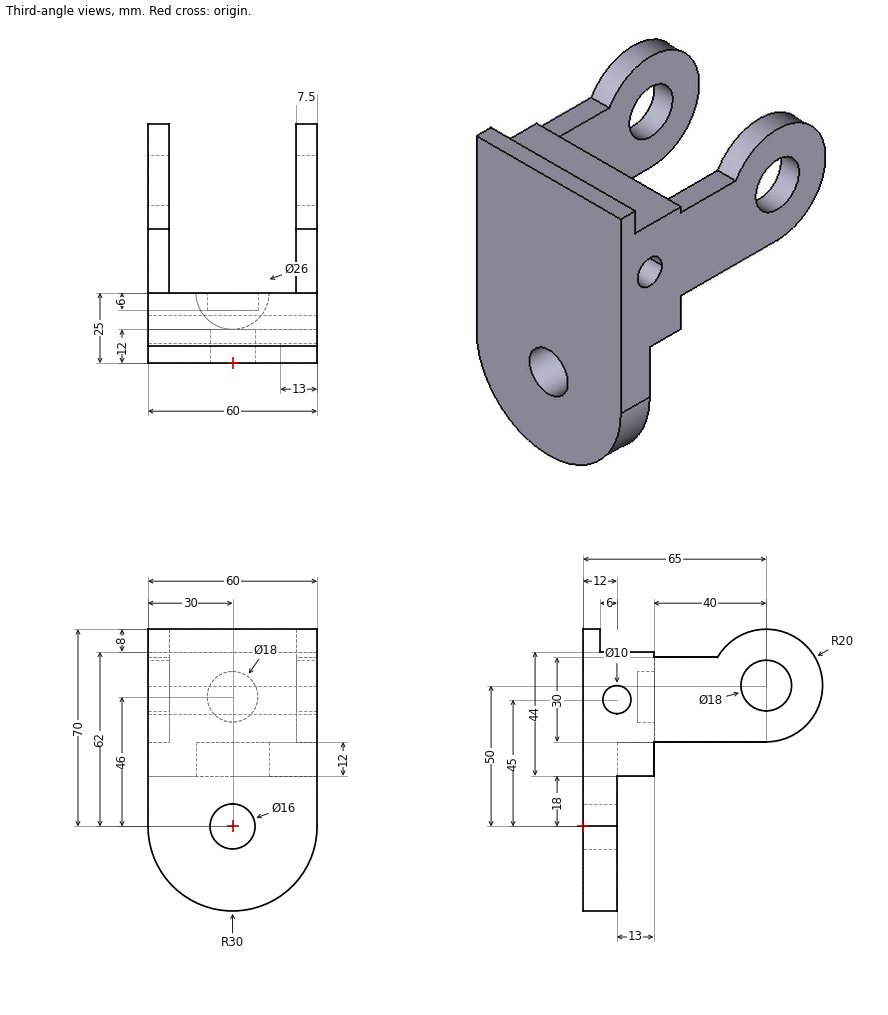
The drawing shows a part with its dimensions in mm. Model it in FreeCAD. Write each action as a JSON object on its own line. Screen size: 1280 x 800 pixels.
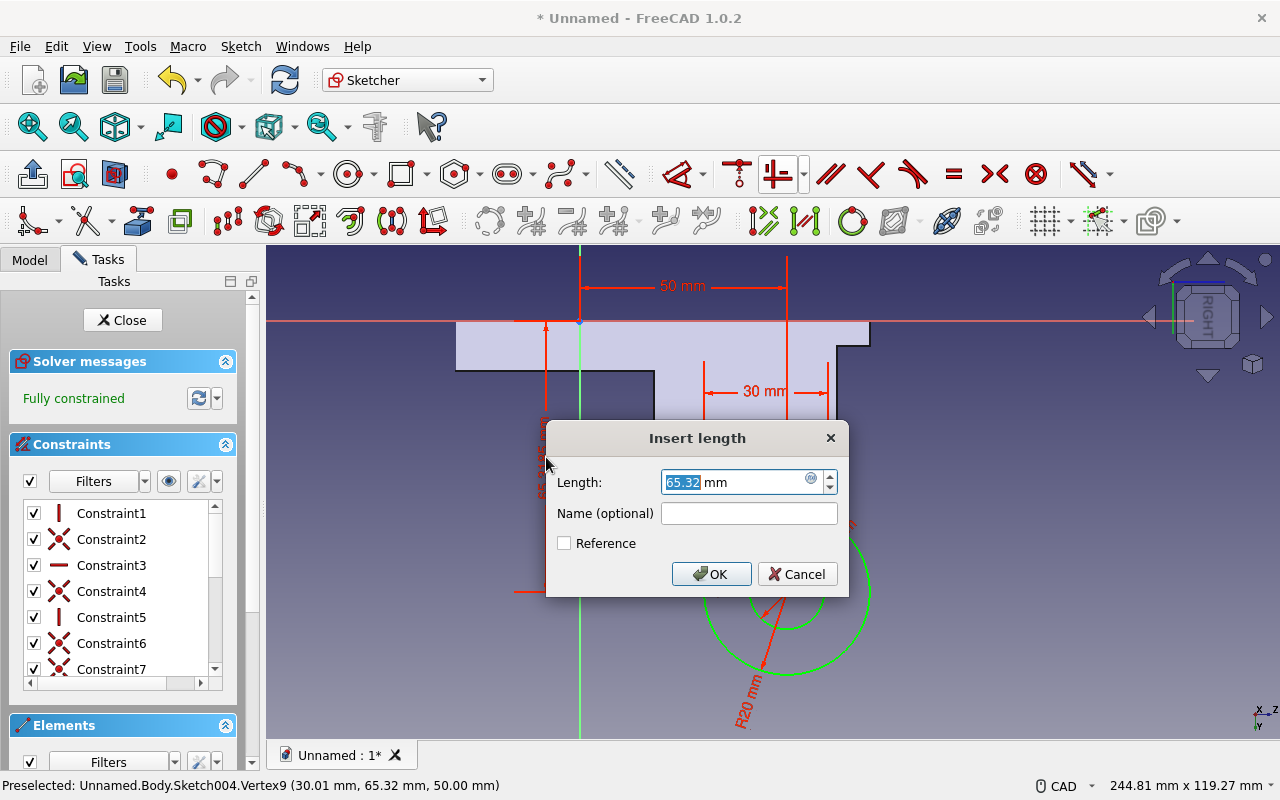
{"action": "type", "text": "65"}
{"action": "key", "text": "Return"}
{"action": "key", "text": "Escape"}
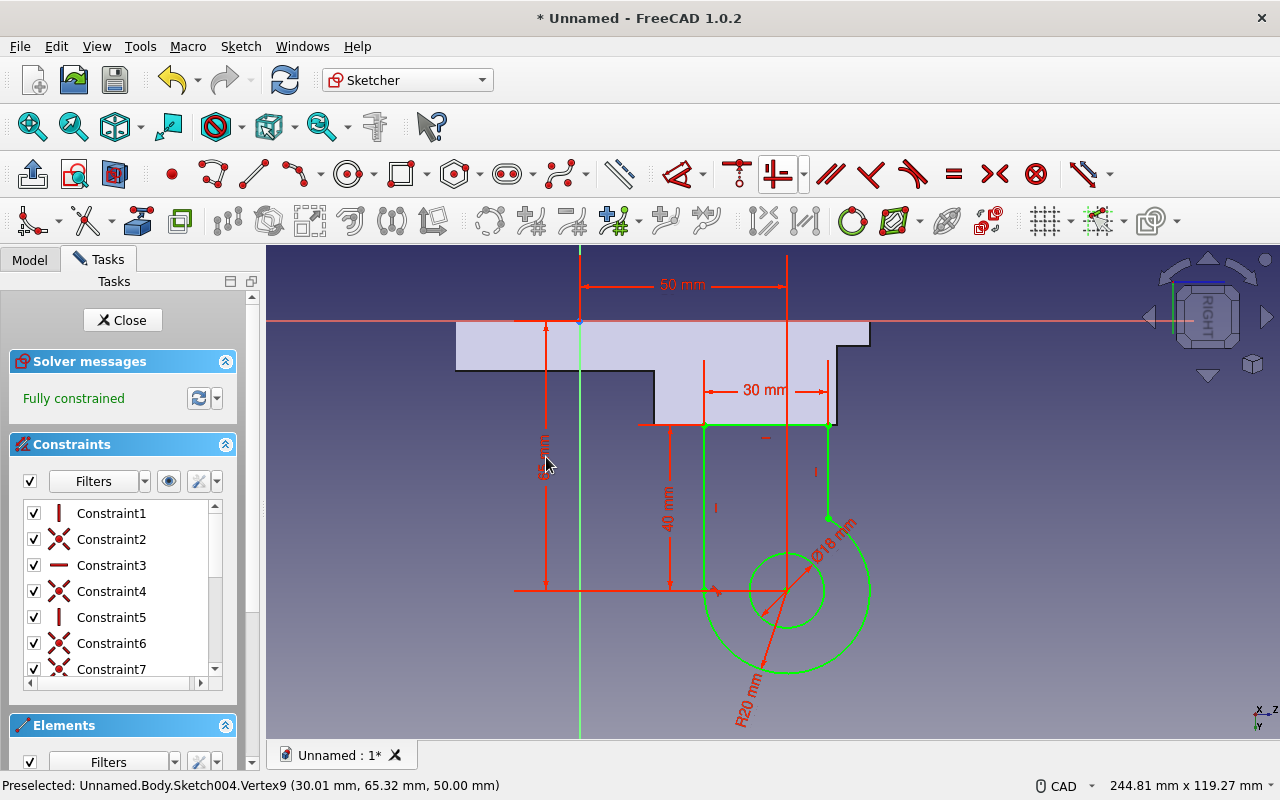
{"action": "left_click", "coordinate": [123, 320]}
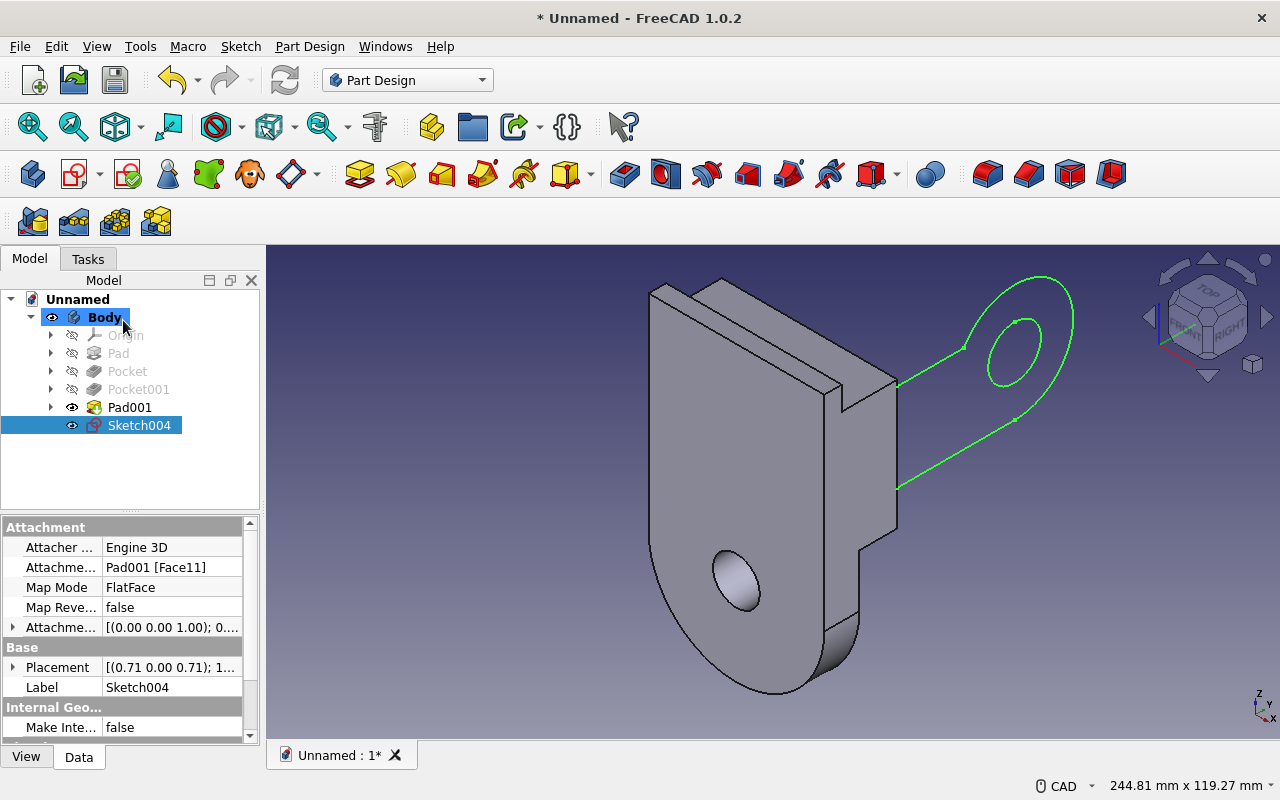
{"action": "left_click", "coordinate": [360, 174]}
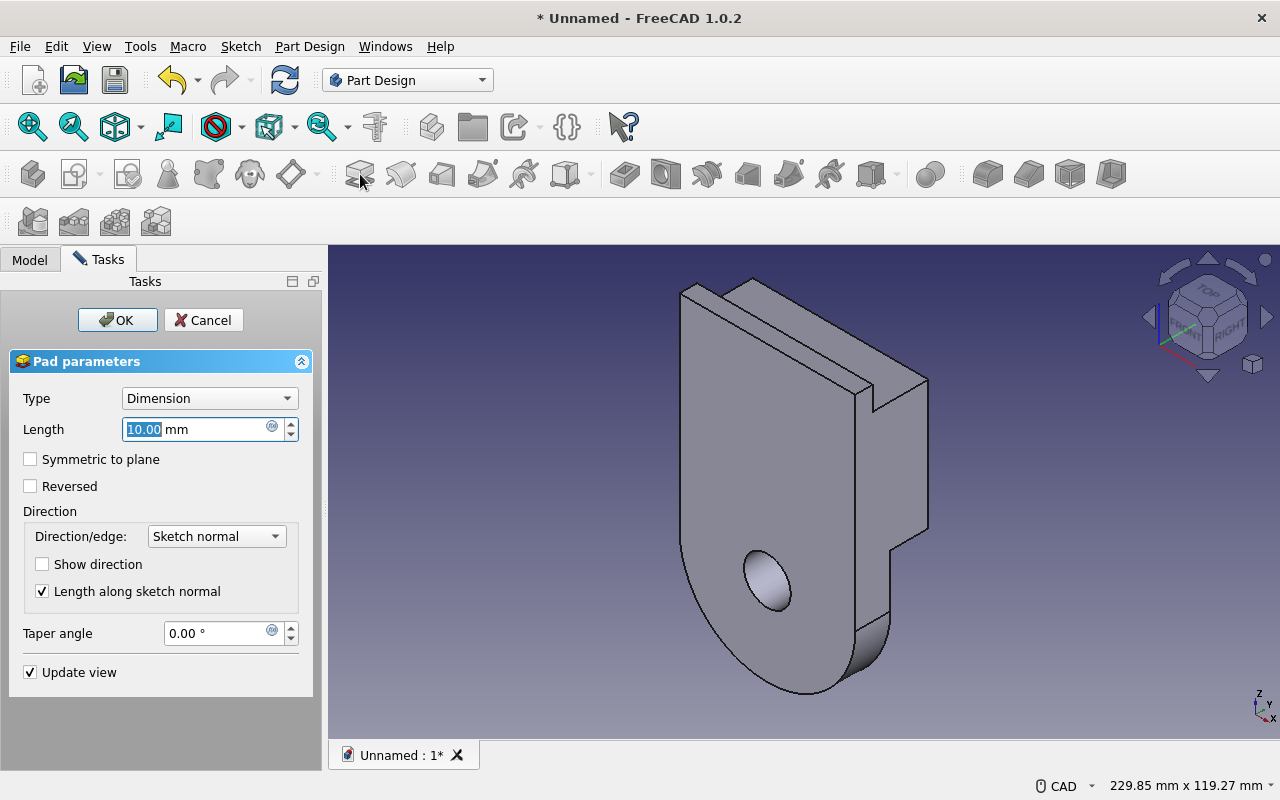
{"action": "type", "text": "7.5"}
{"action": "key", "text": "Tab"}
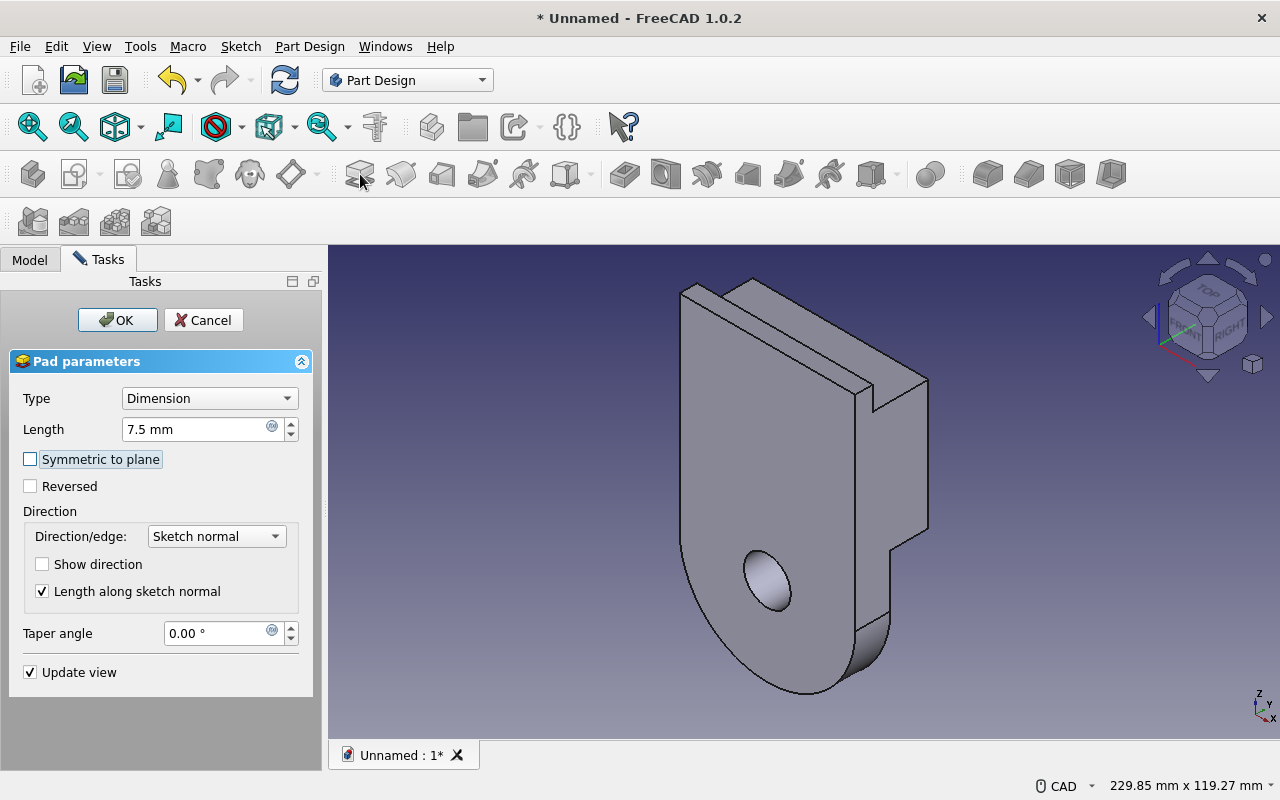
{"action": "left_click", "coordinate": [31, 486]}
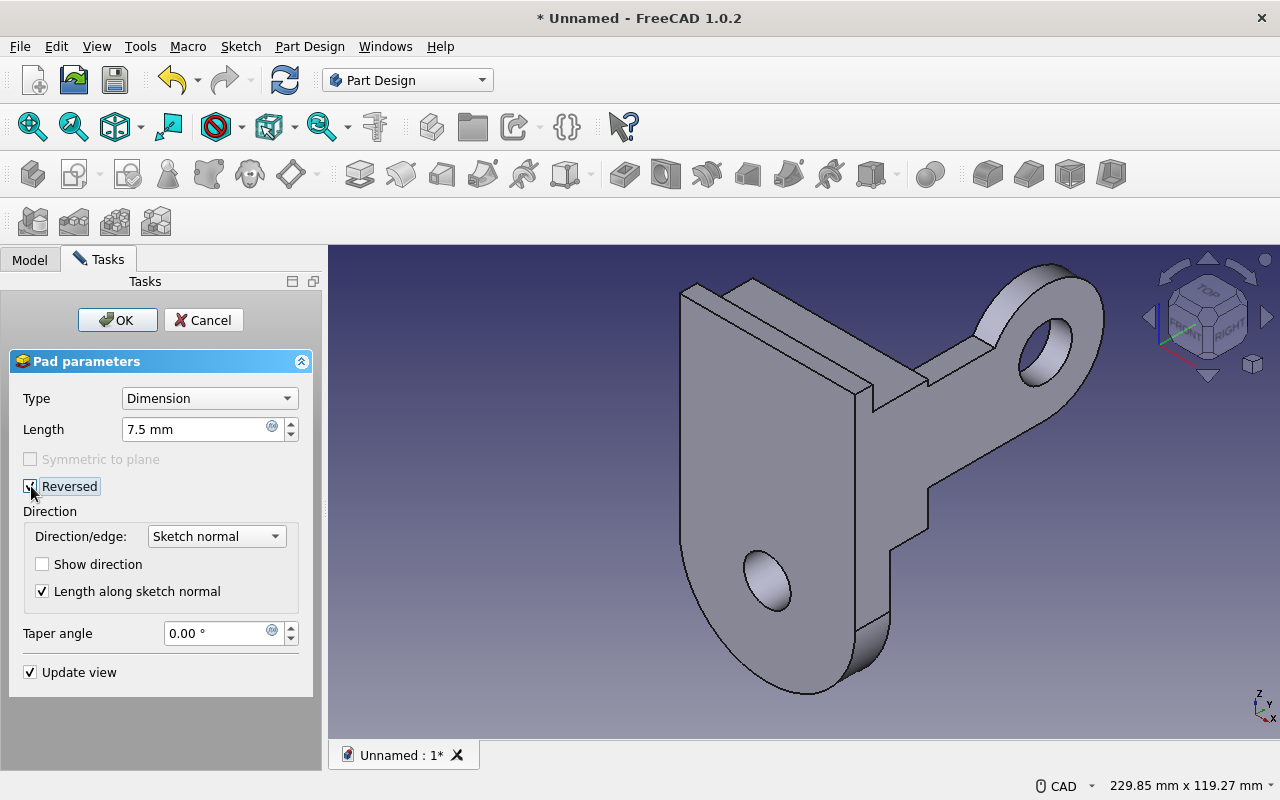
{"action": "left_click", "coordinate": [118, 320]}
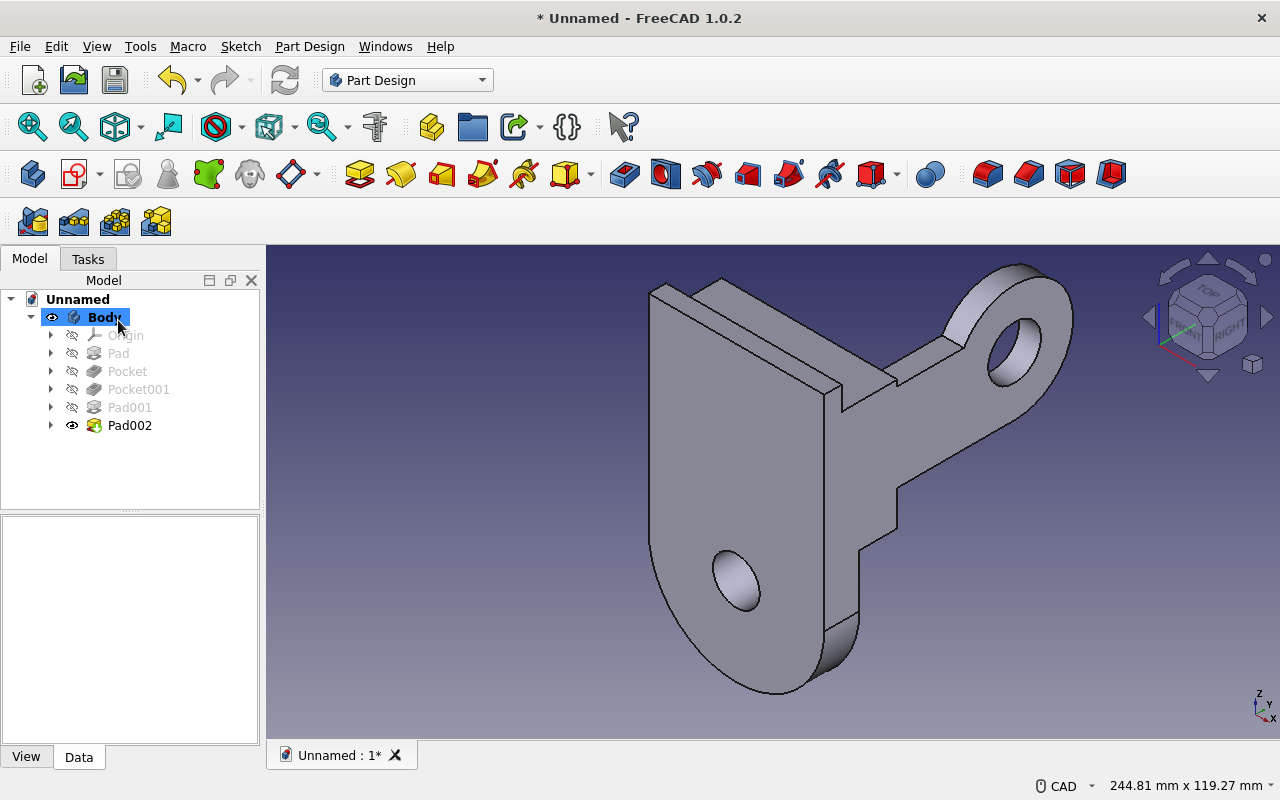
{"action": "key", "text": "v f"}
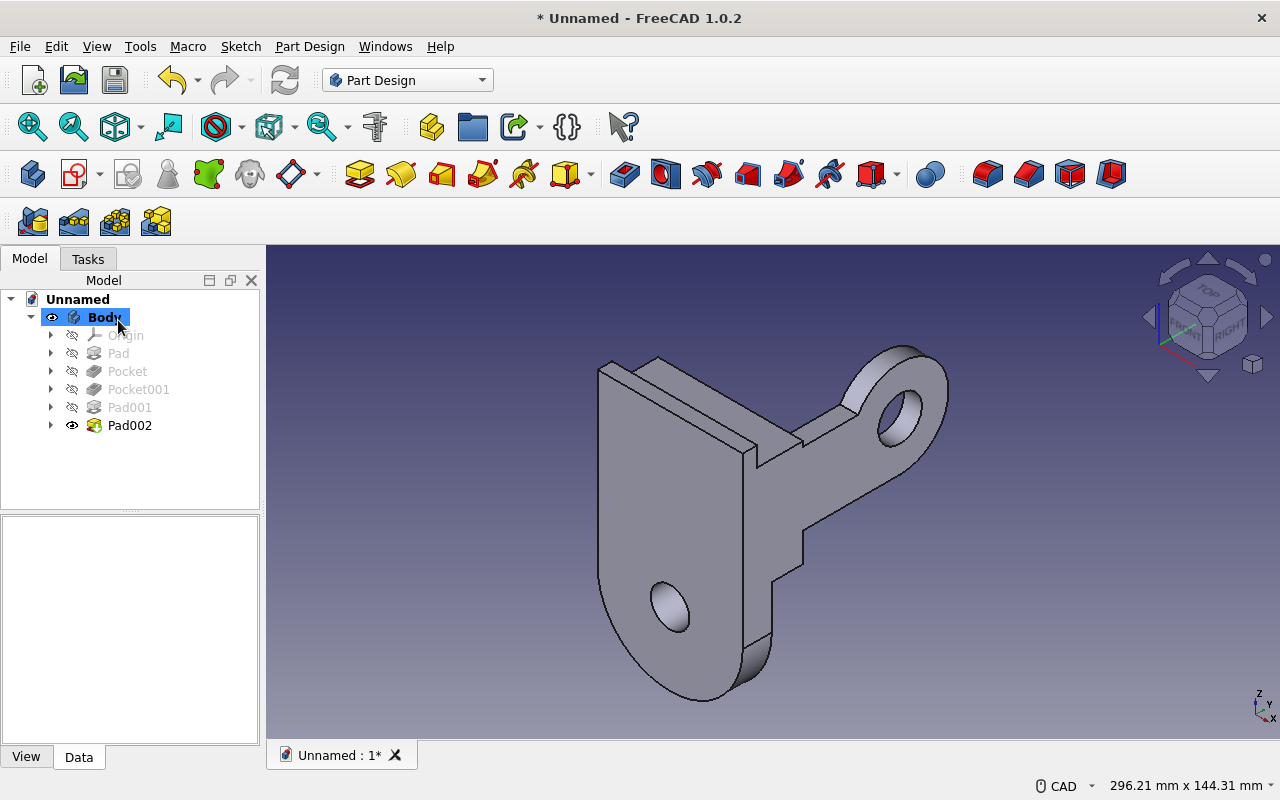
{"action": "left_click", "coordinate": [117, 425]}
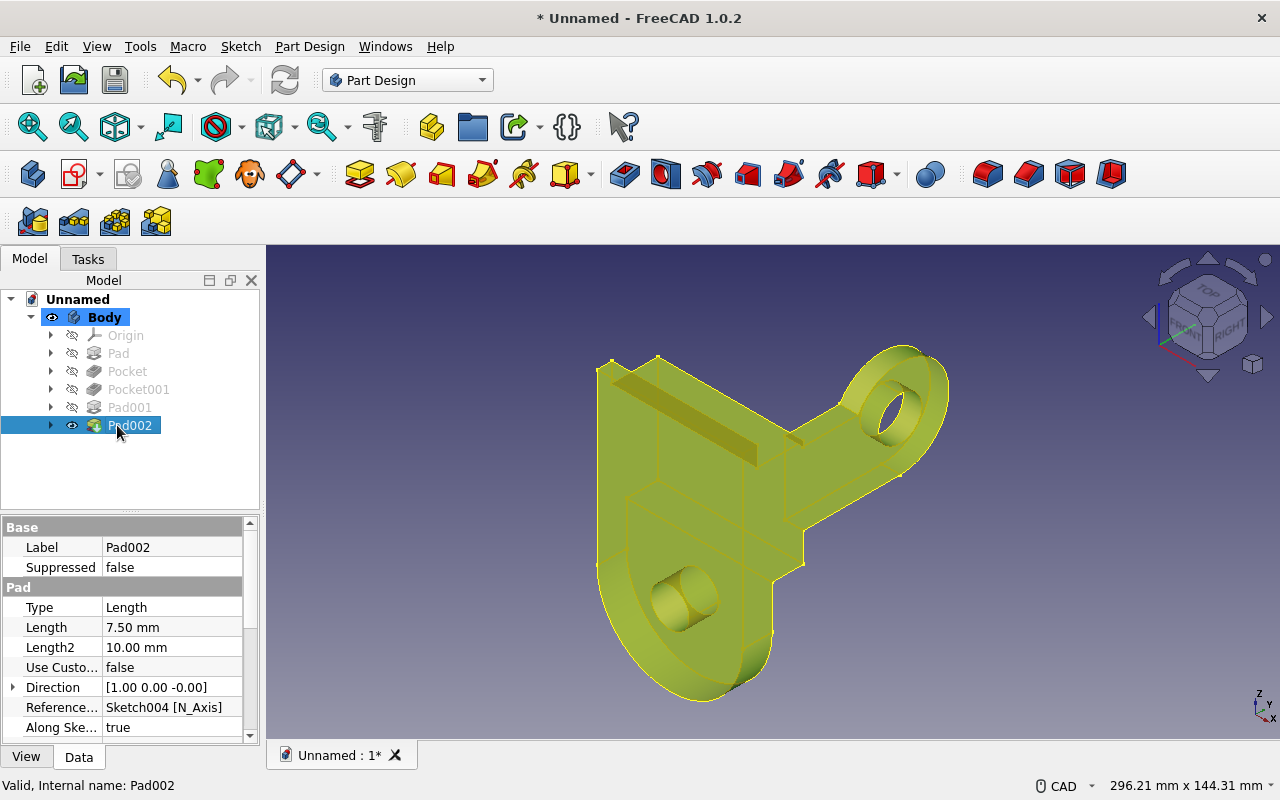
{"action": "left_click", "coordinate": [33, 222]}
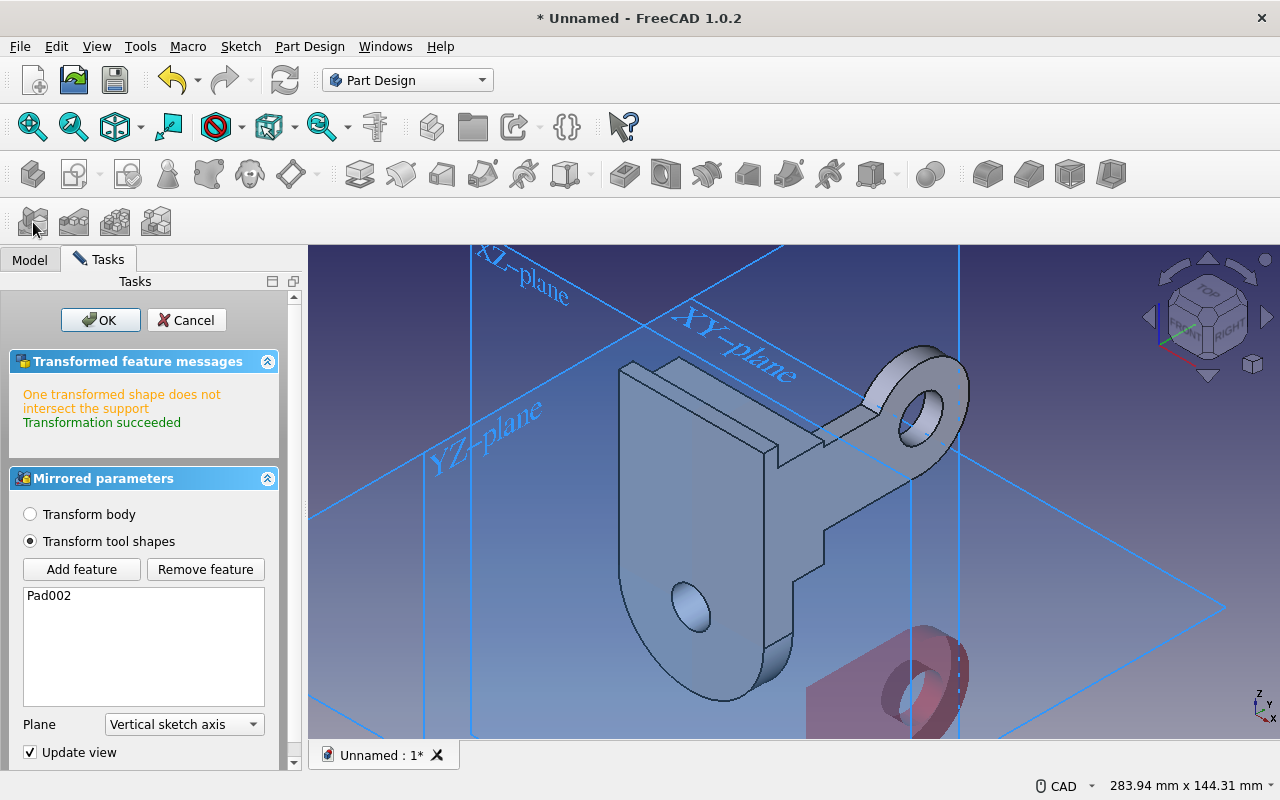
{"action": "left_click", "coordinate": [185, 724]}